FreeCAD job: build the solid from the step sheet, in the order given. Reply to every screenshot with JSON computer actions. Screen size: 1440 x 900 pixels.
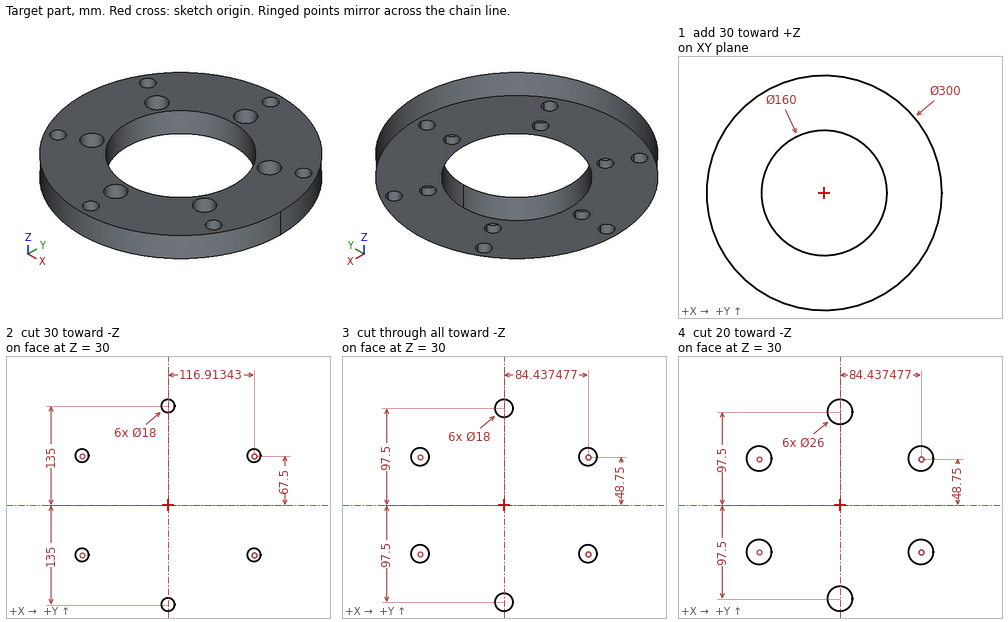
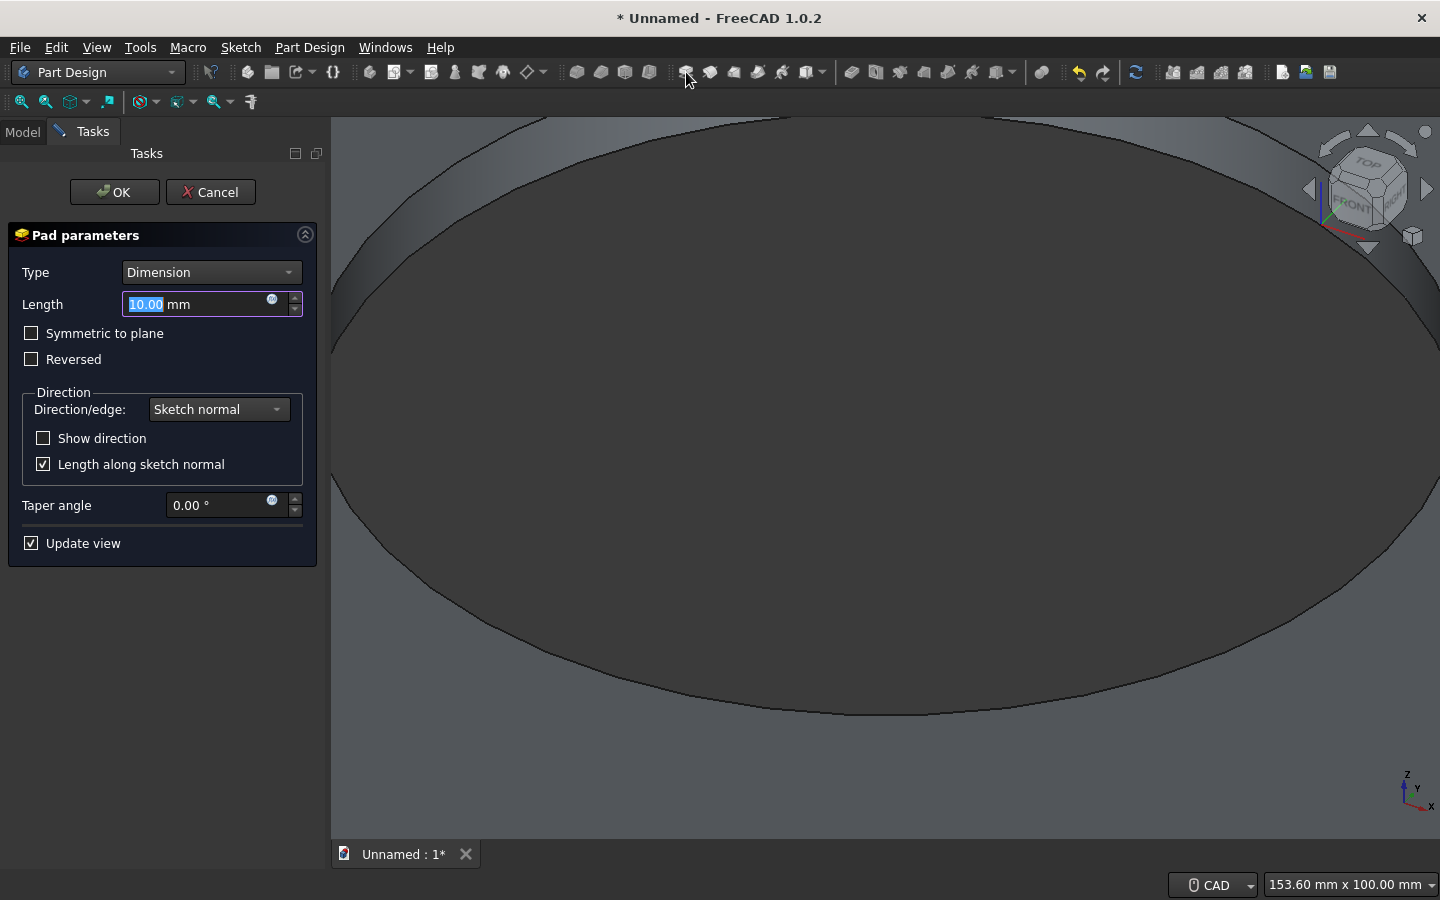
{"action": "type", "text": "30"}
{"action": "key", "text": "Tab"}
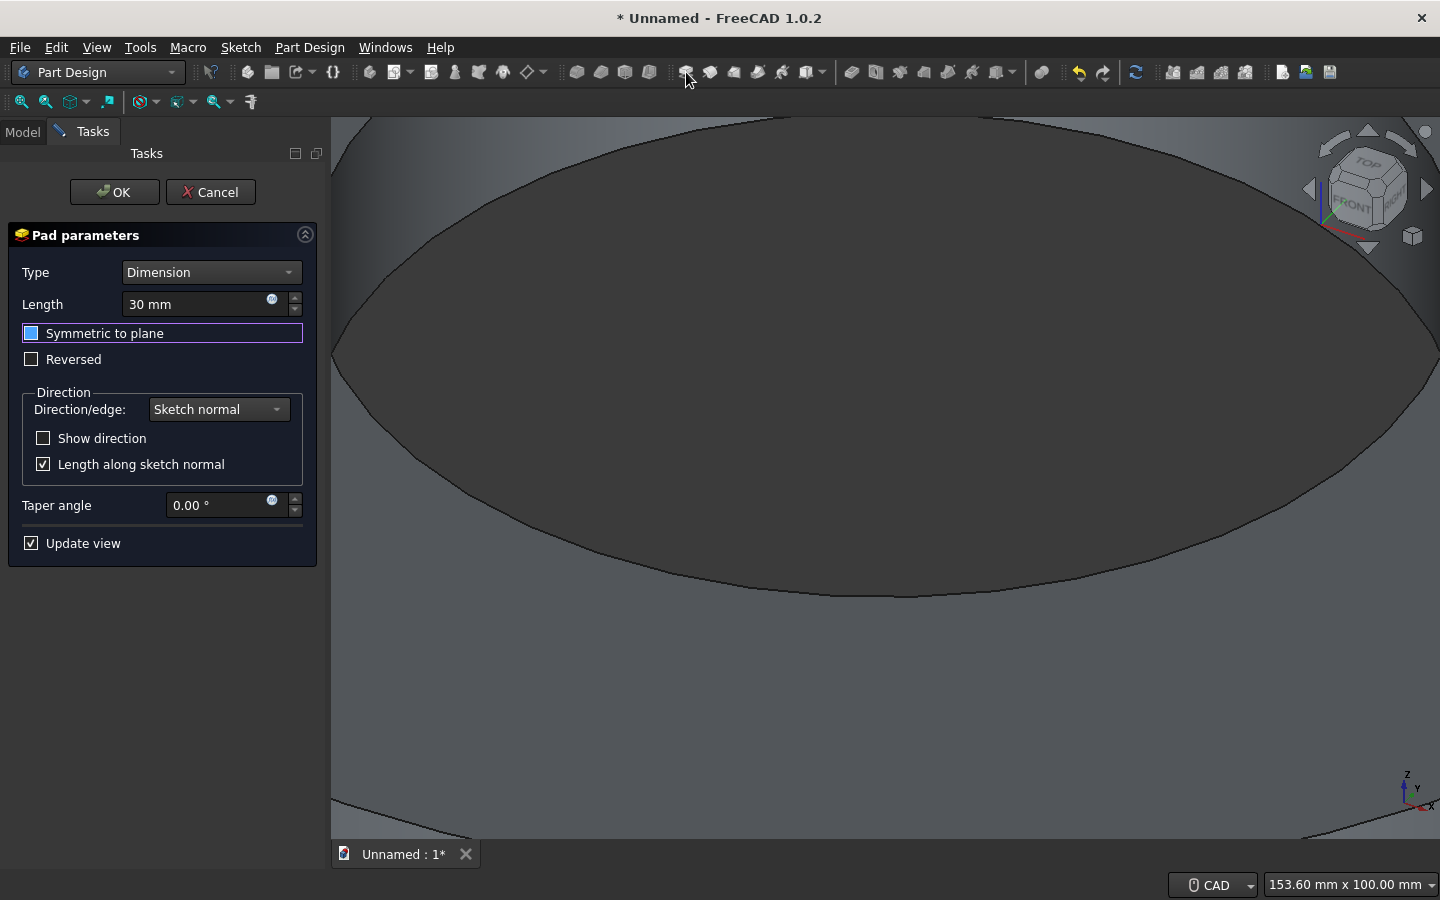
{"action": "left_click", "coordinate": [115, 192]}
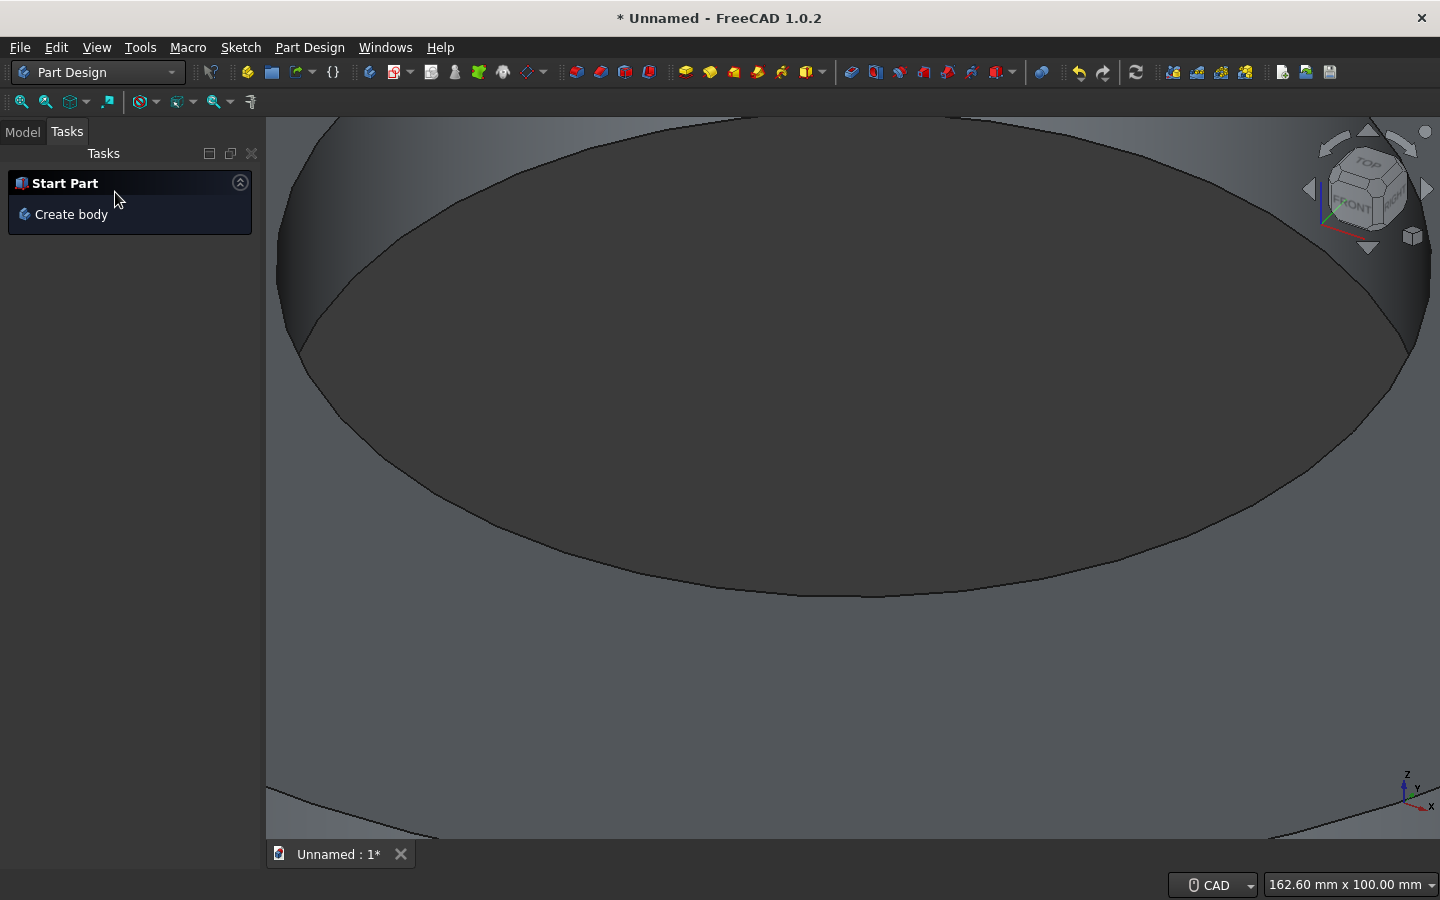
{"action": "key", "text": "v f"}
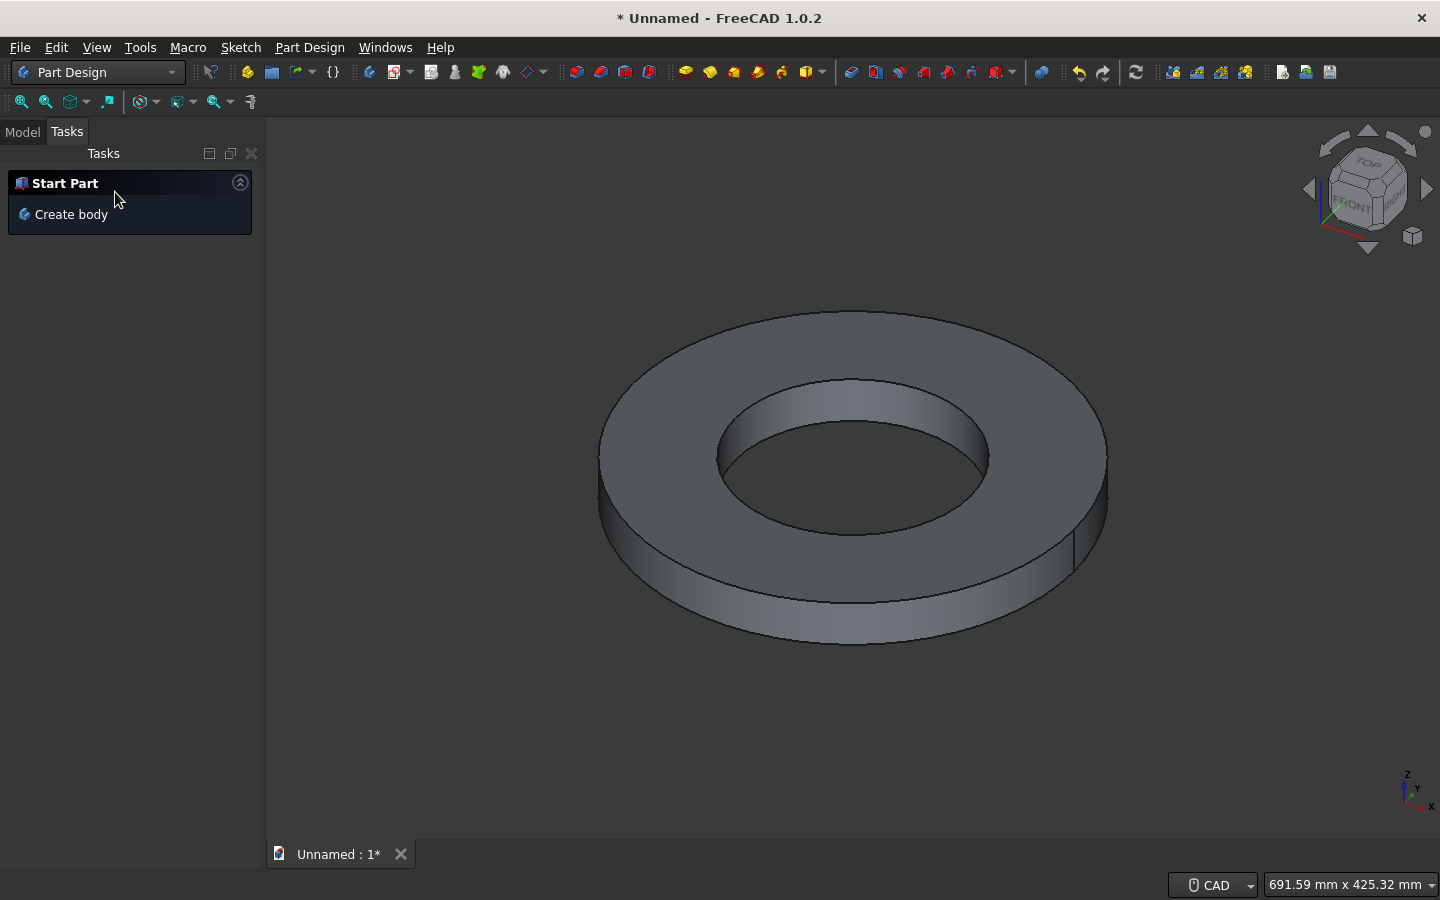
{"action": "left_click", "coordinate": [906, 570]}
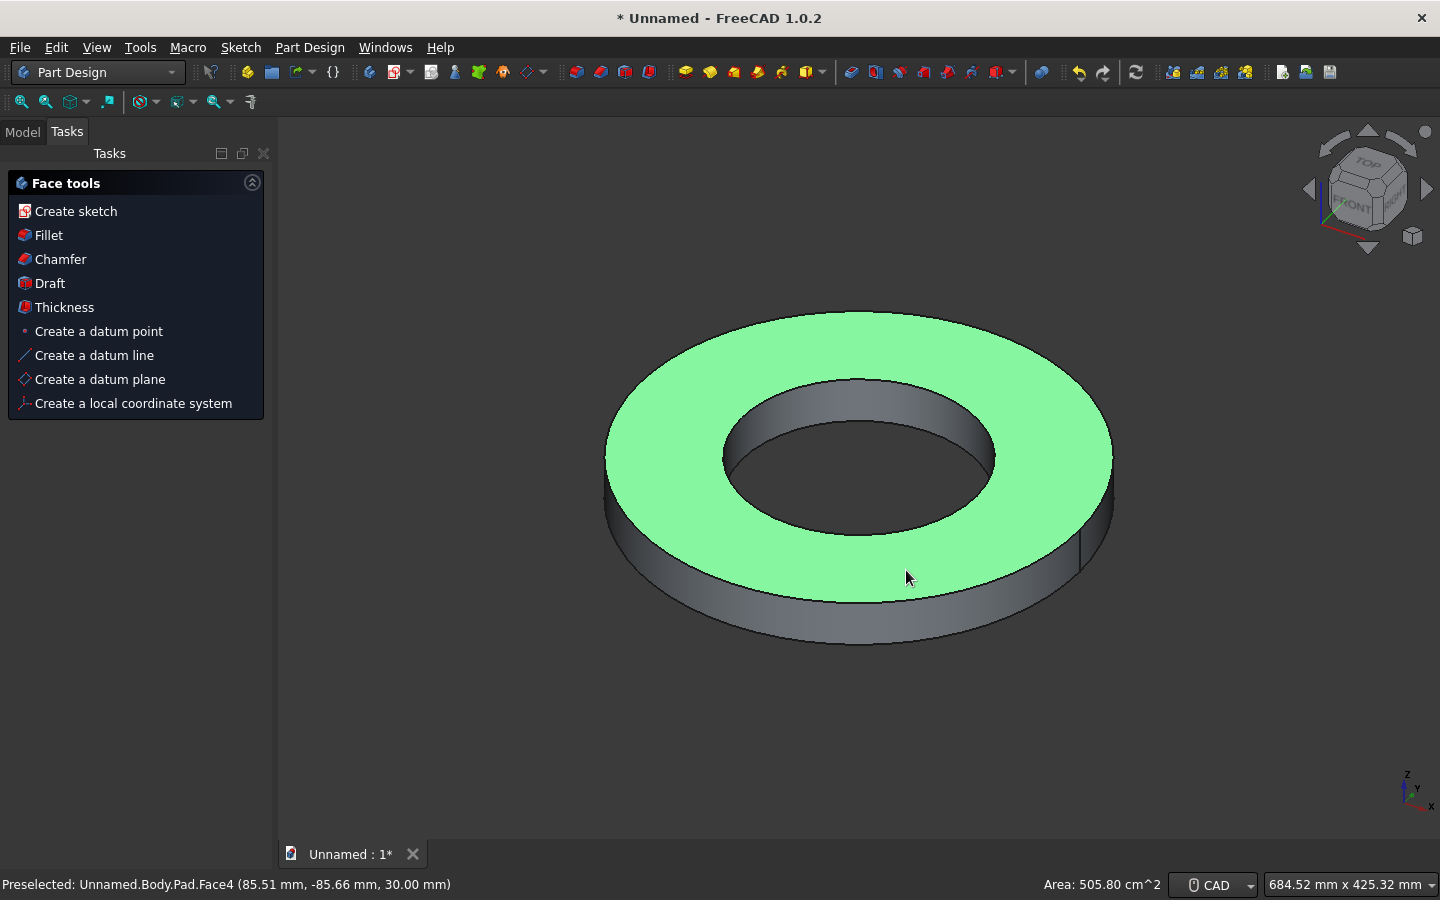
{"action": "left_click", "coordinate": [394, 72]}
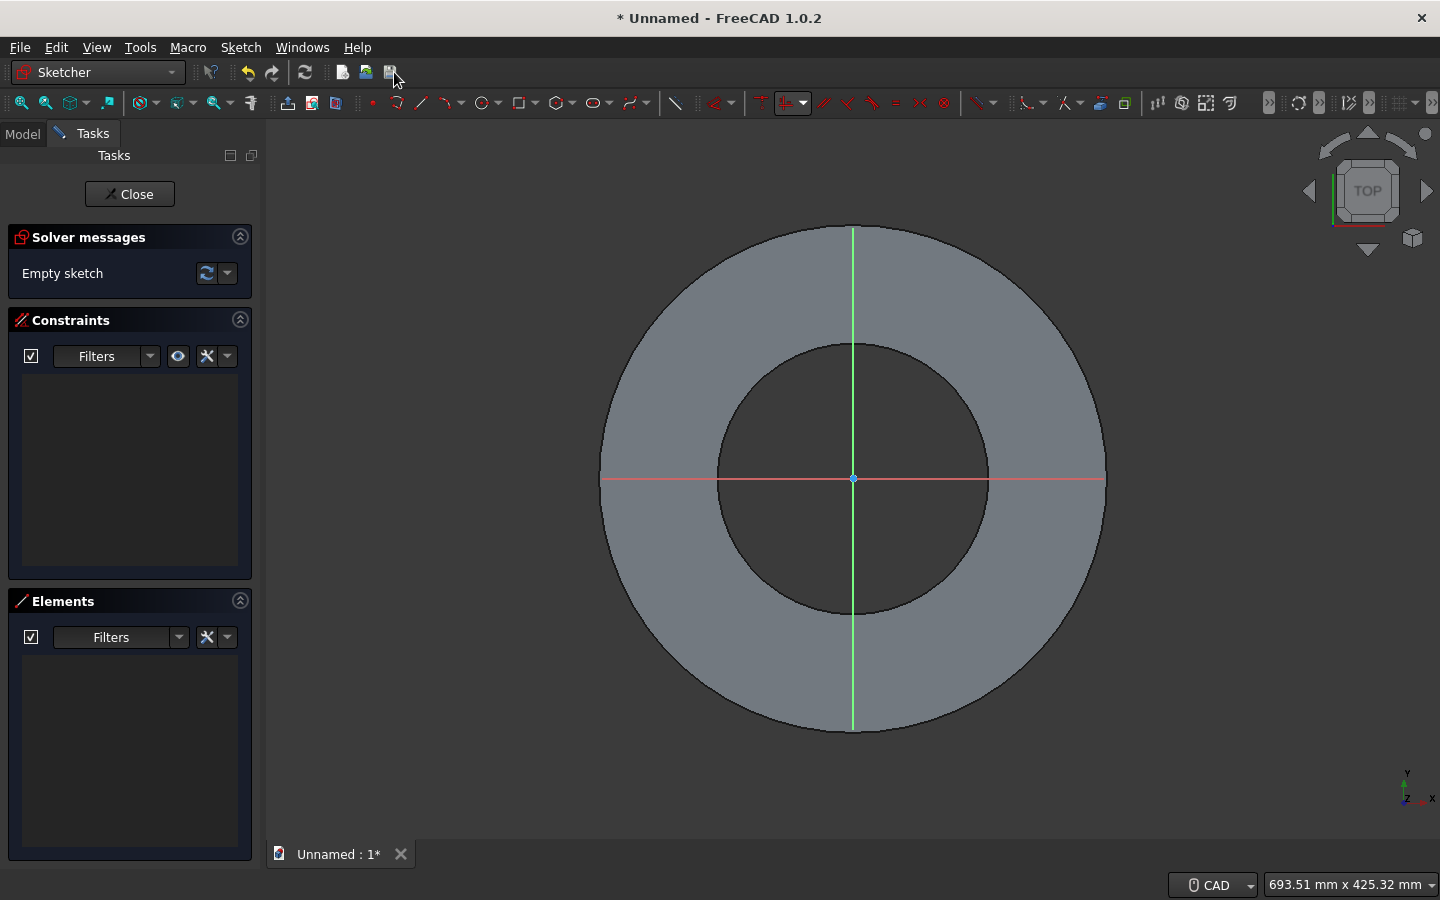
{"action": "key", "text": "g c"}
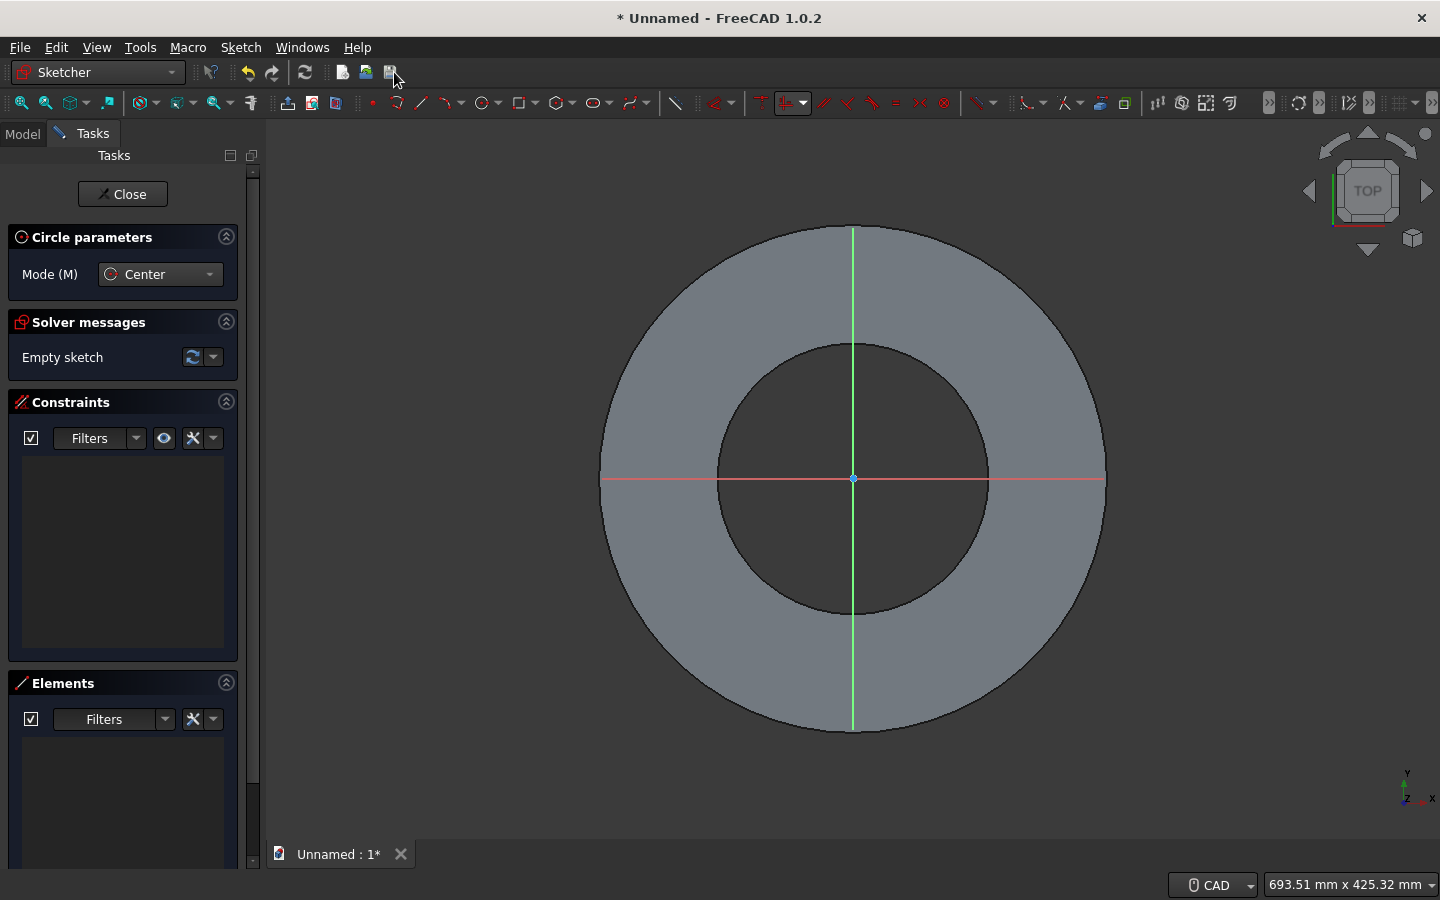
{"action": "scroll", "coordinate": [853, 250], "scroll_direction": "up", "scroll_amount": 2}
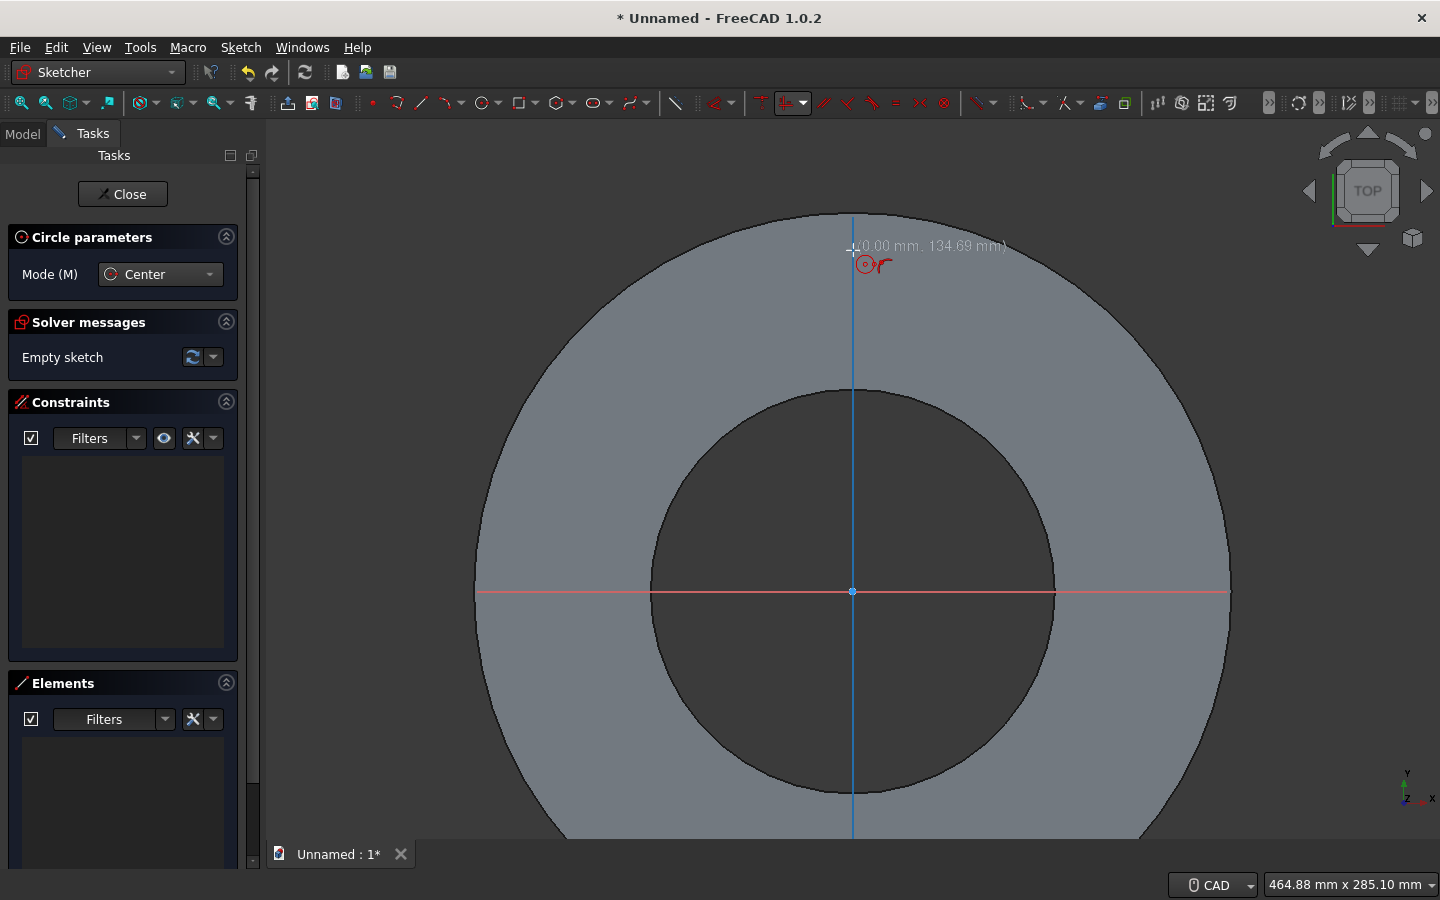
{"action": "left_click", "coordinate": [853, 251]}
{"action": "left_click", "coordinate": [869, 235]}